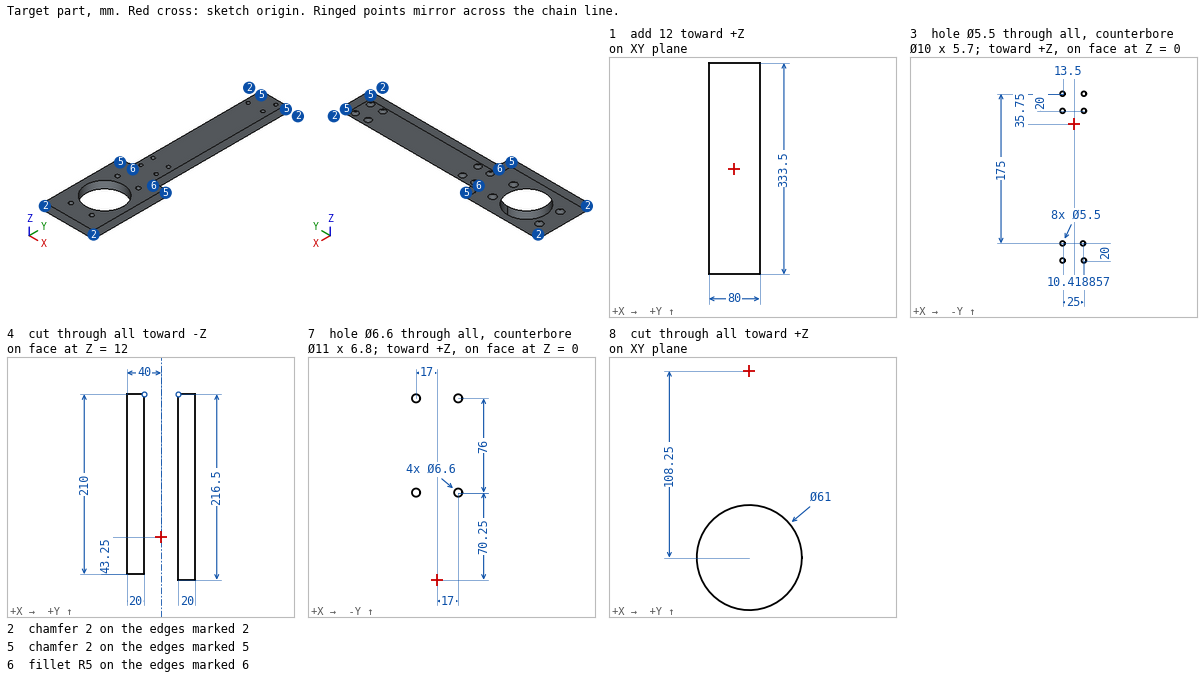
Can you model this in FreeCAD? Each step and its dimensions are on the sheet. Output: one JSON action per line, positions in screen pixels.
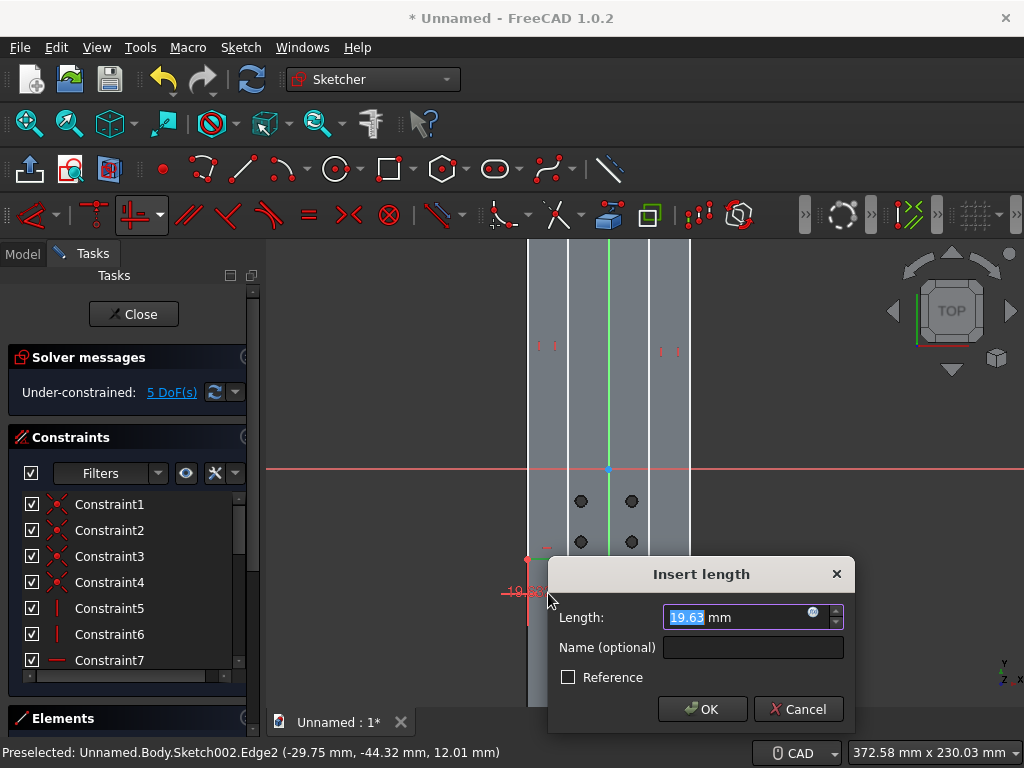
{"action": "type", "text": "20"}
{"action": "key", "text": "Return"}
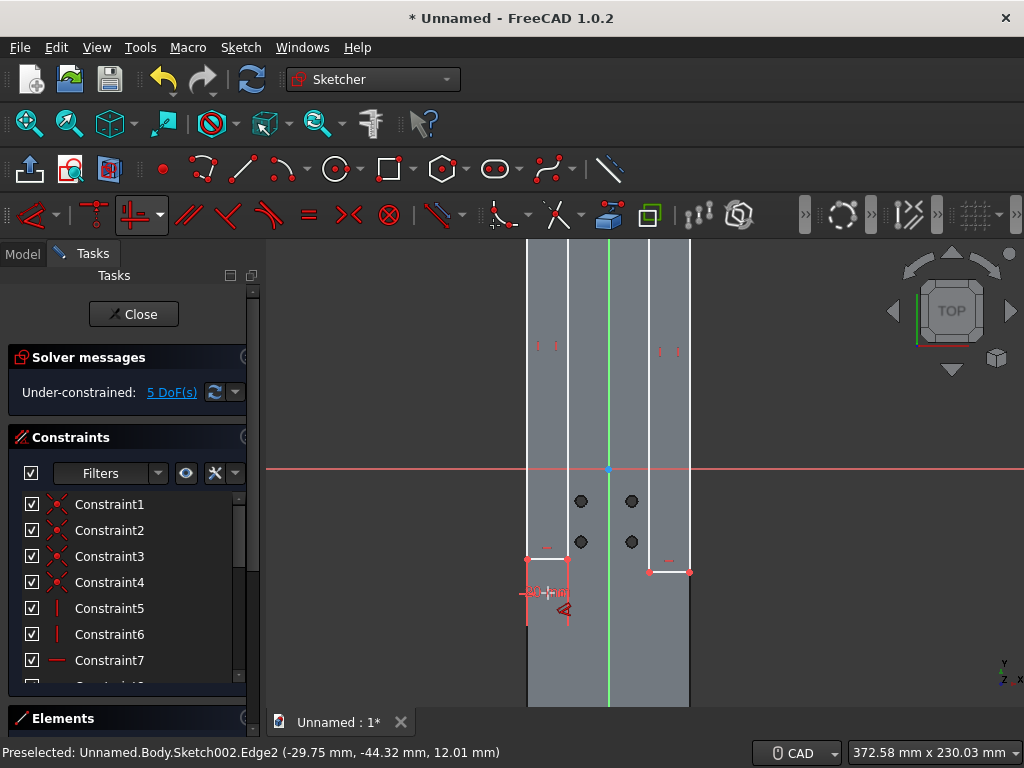
{"action": "left_click", "coordinate": [661, 572]}
{"action": "left_click", "coordinate": [670, 606]}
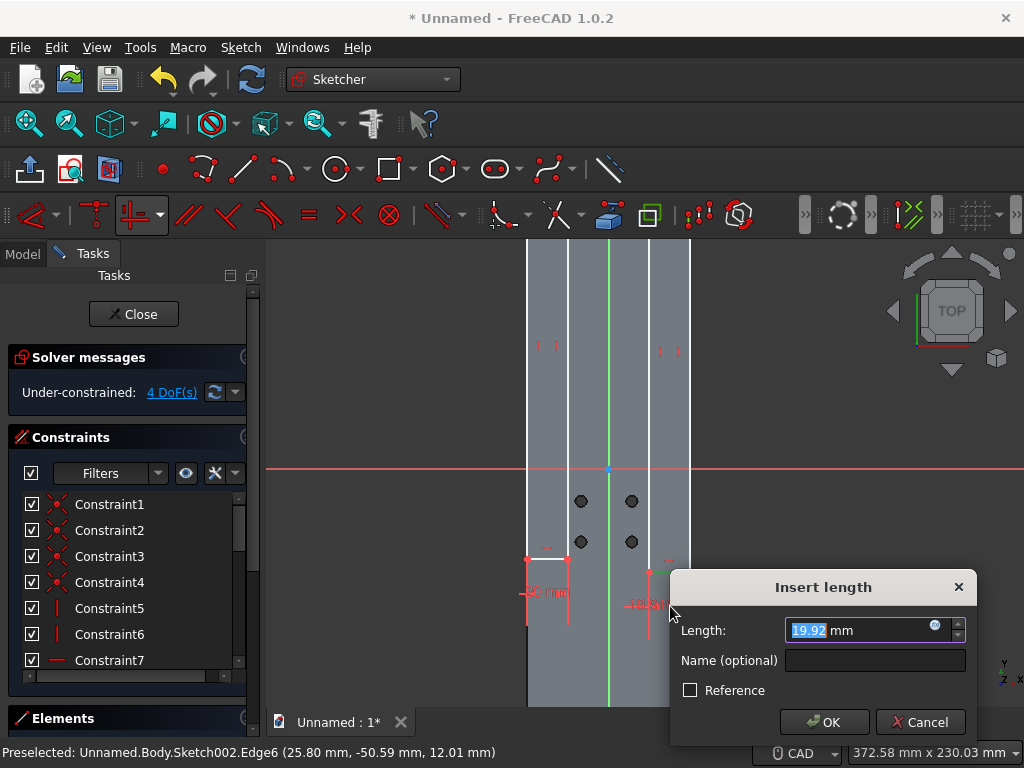
{"action": "type", "text": "20"}
{"action": "key", "text": "Return"}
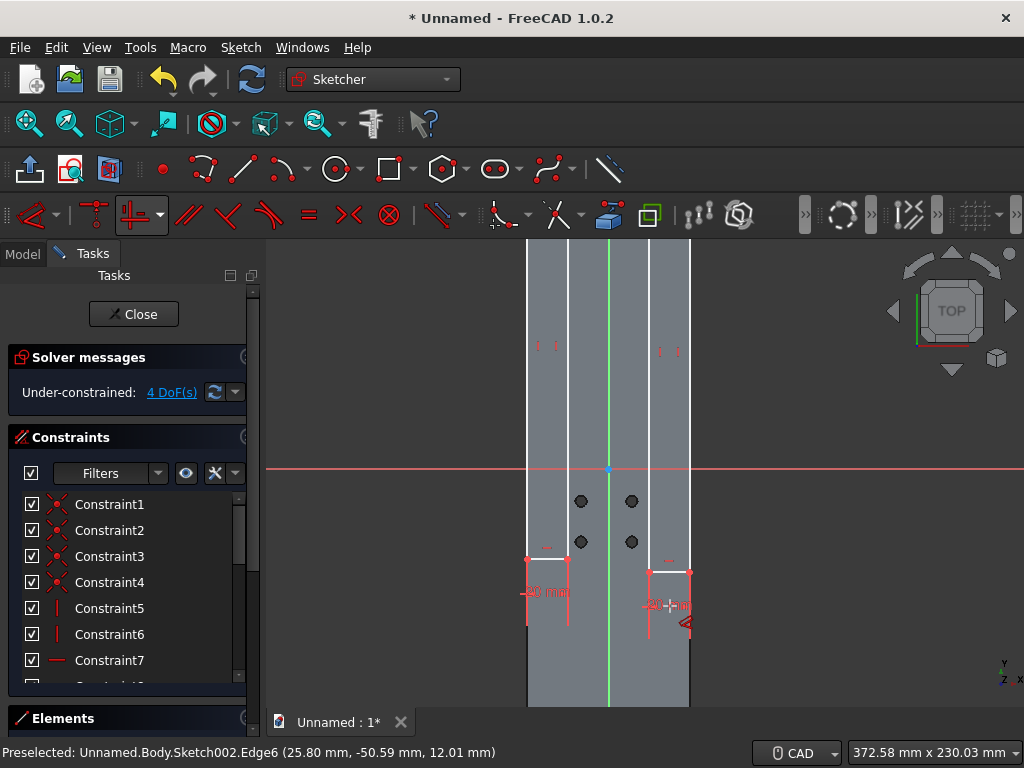
{"action": "left_click", "coordinate": [527, 431]}
{"action": "left_click", "coordinate": [493, 413]}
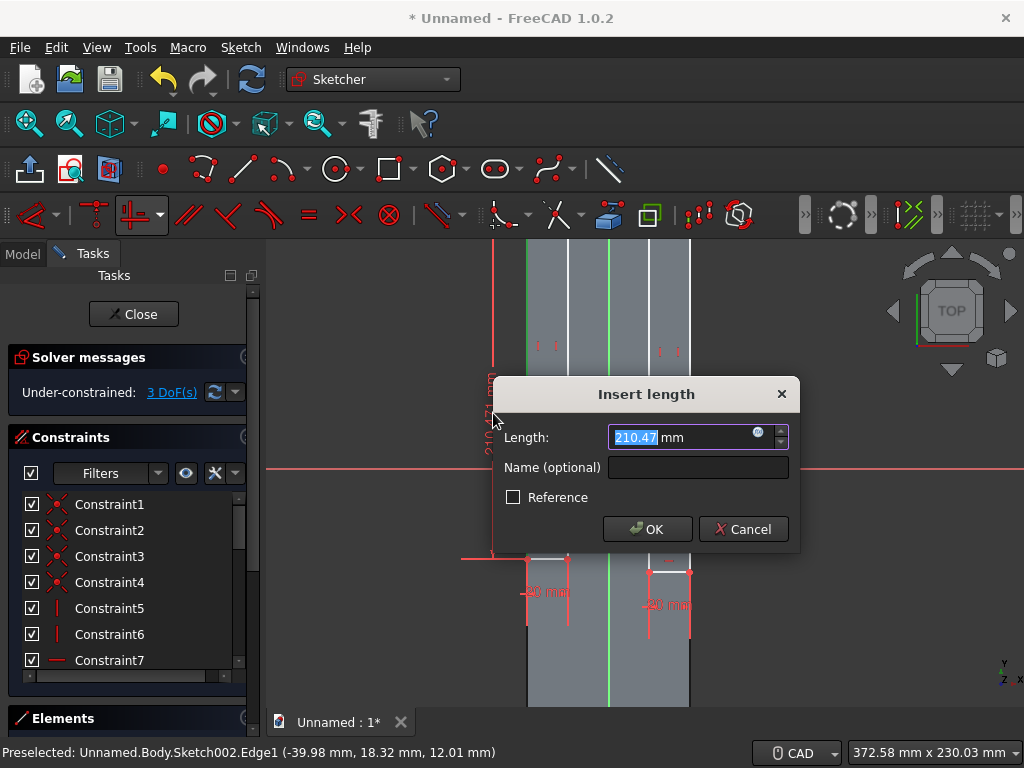
{"action": "type", "text": "210"}
{"action": "key", "text": "Return"}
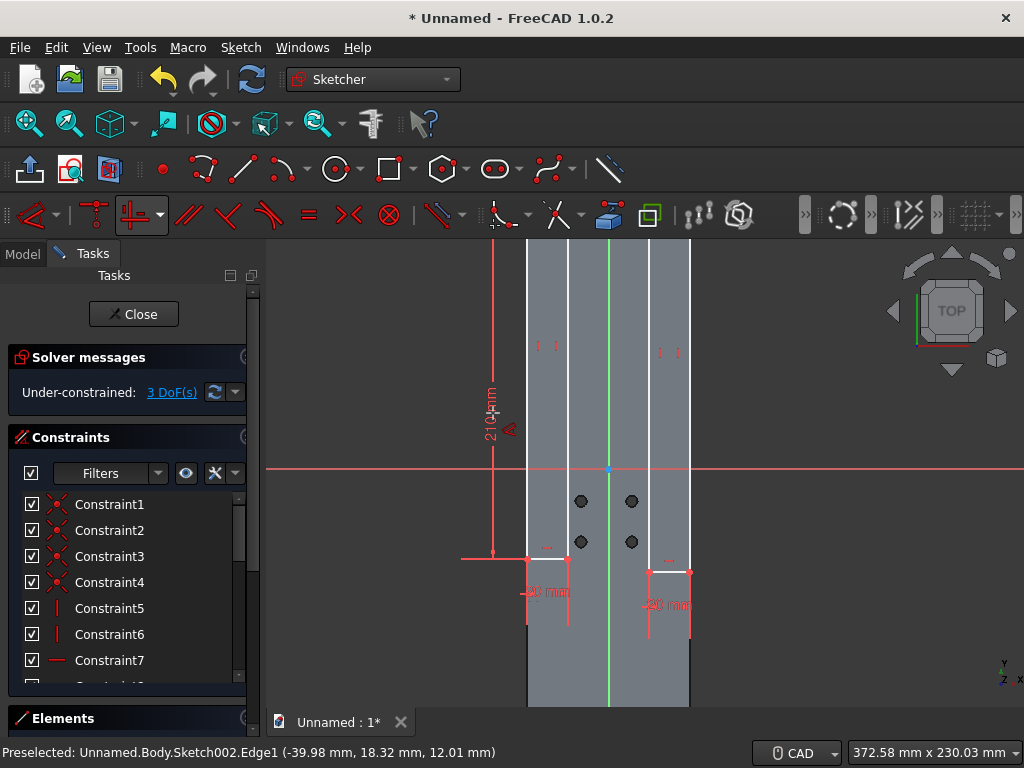
{"action": "scroll", "coordinate": [511, 679], "scroll_direction": "down", "scroll_amount": 2}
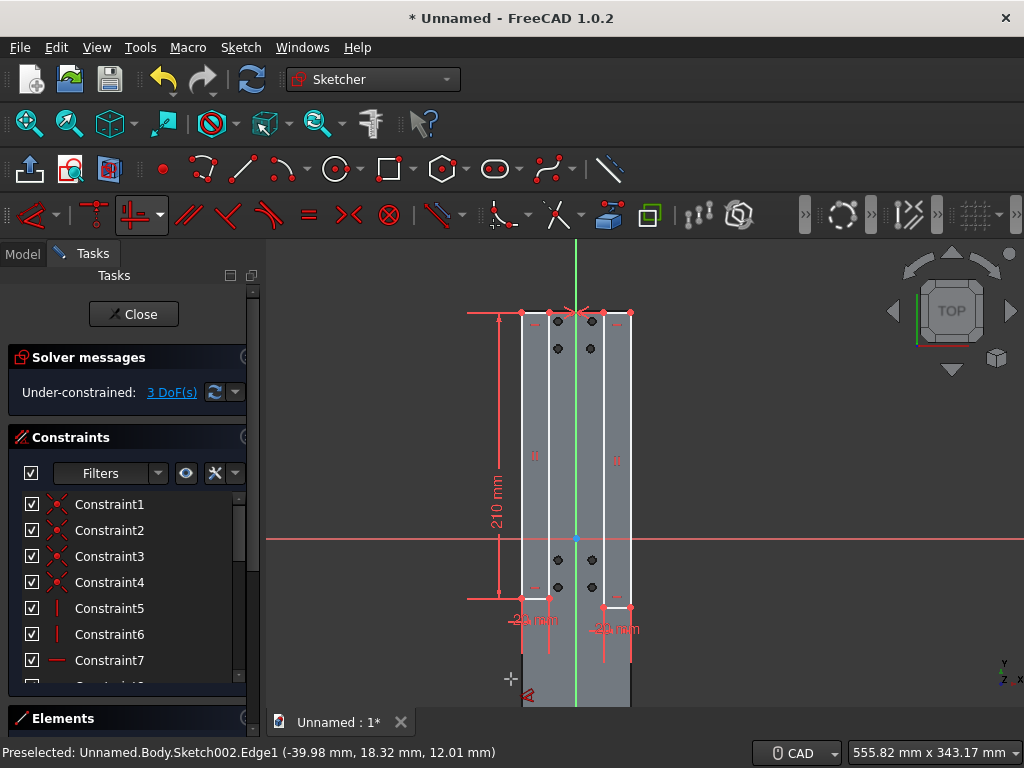
{"action": "left_click", "coordinate": [522, 313]}
{"action": "left_click", "coordinate": [549, 279]}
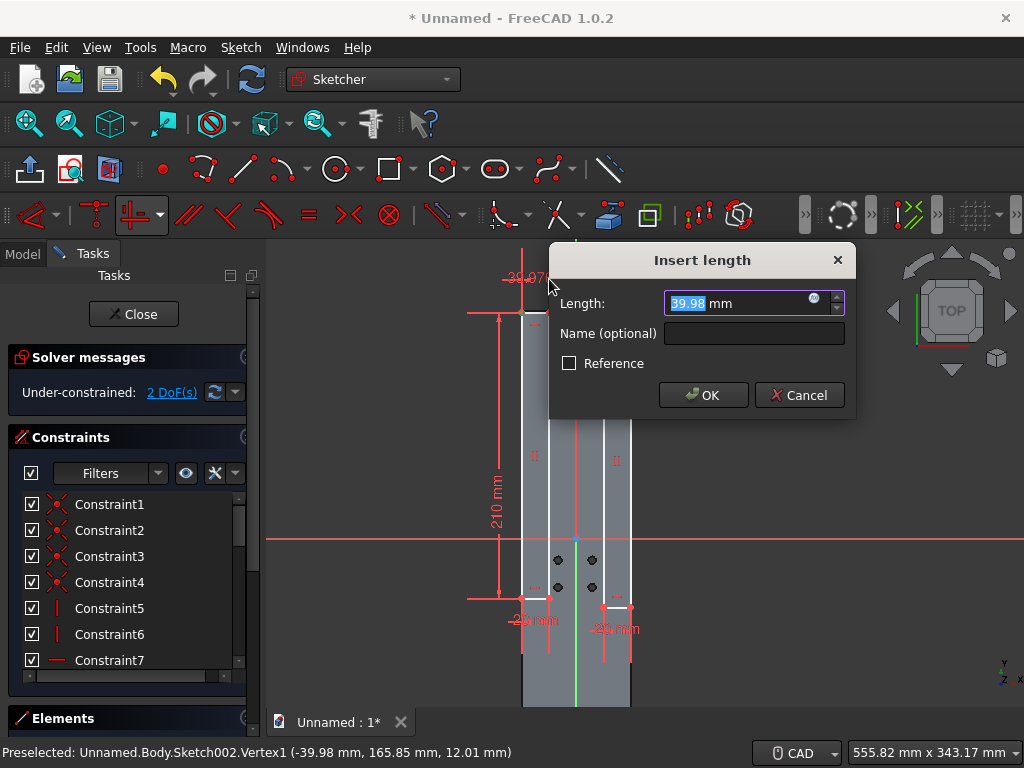
{"action": "type", "text": "40"}
{"action": "key", "text": "Return"}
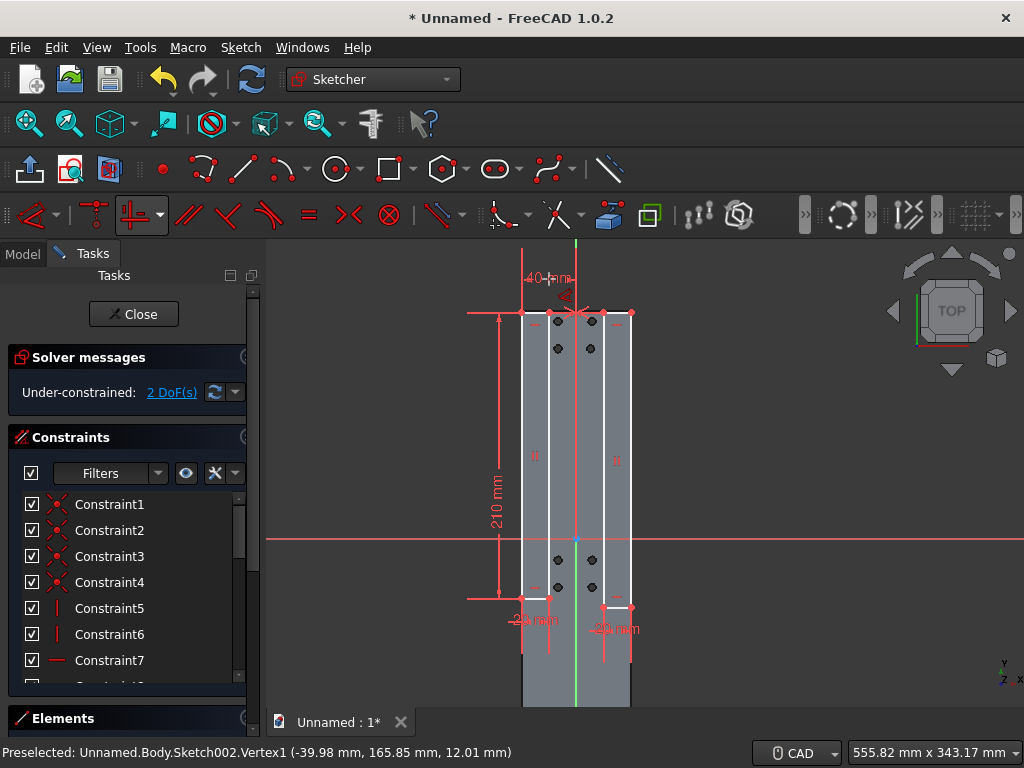
{"action": "left_click", "coordinate": [604, 401]}
{"action": "left_click", "coordinate": [662, 460]}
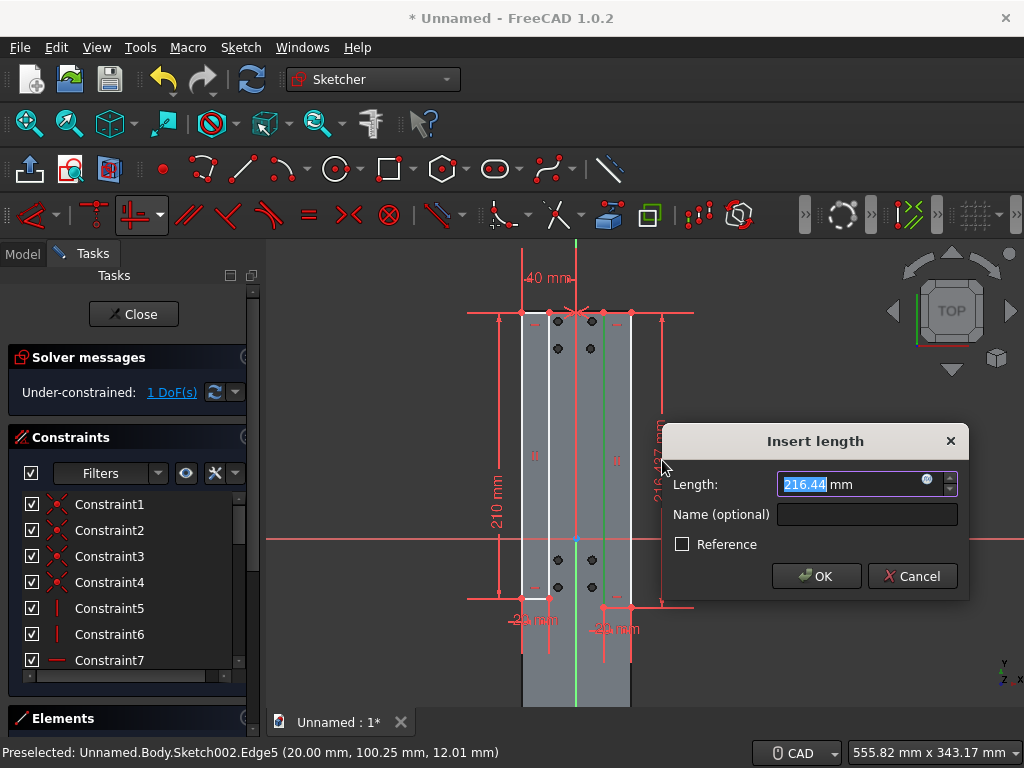
{"action": "type", "text": "216.5"}
{"action": "key", "text": "Return"}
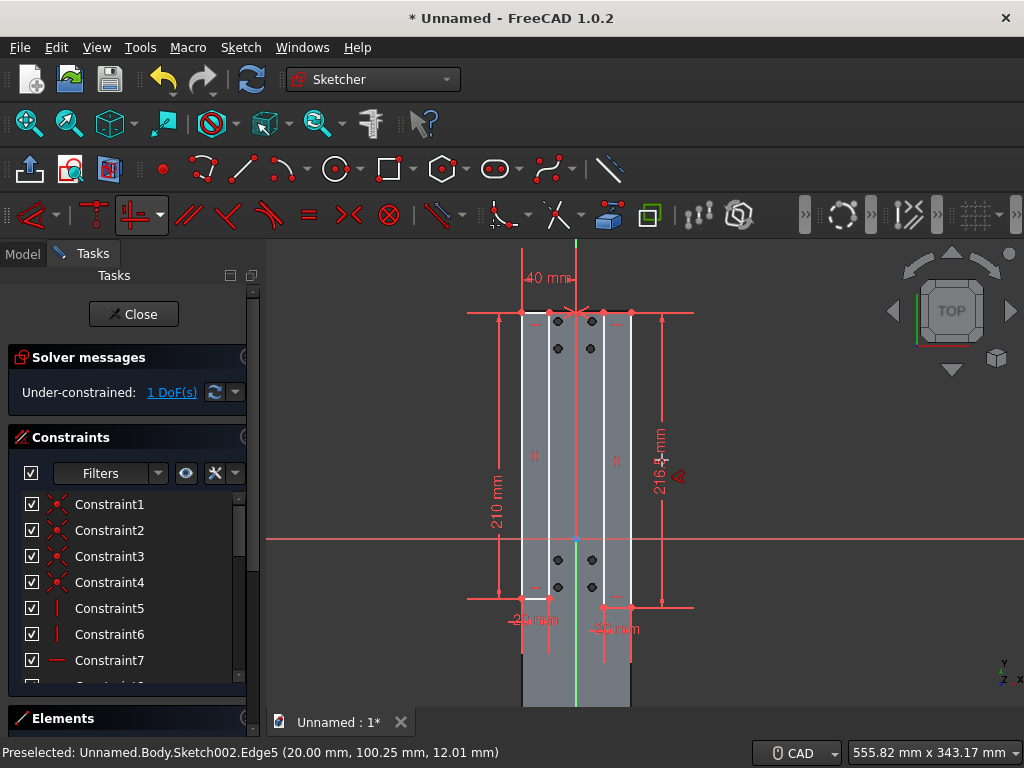
{"action": "left_click", "coordinate": [522, 599]}
{"action": "left_click", "coordinate": [488, 569]}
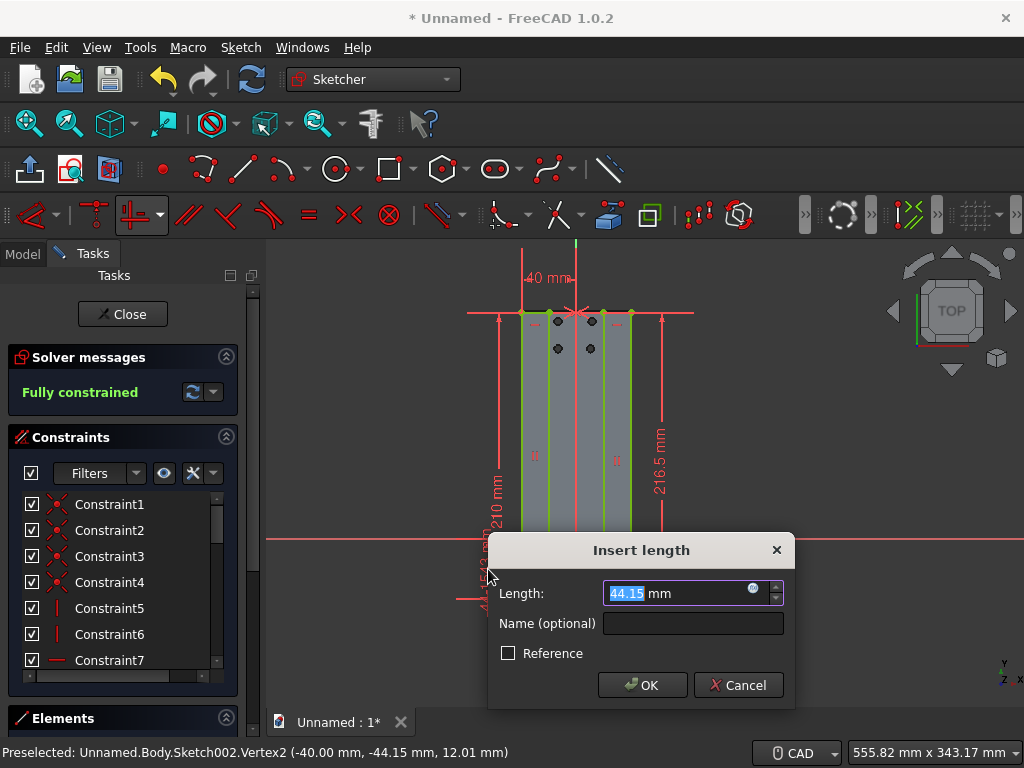
{"action": "type", "text": "43.25"}
{"action": "key", "text": "Return"}
{"action": "key", "text": "Escape"}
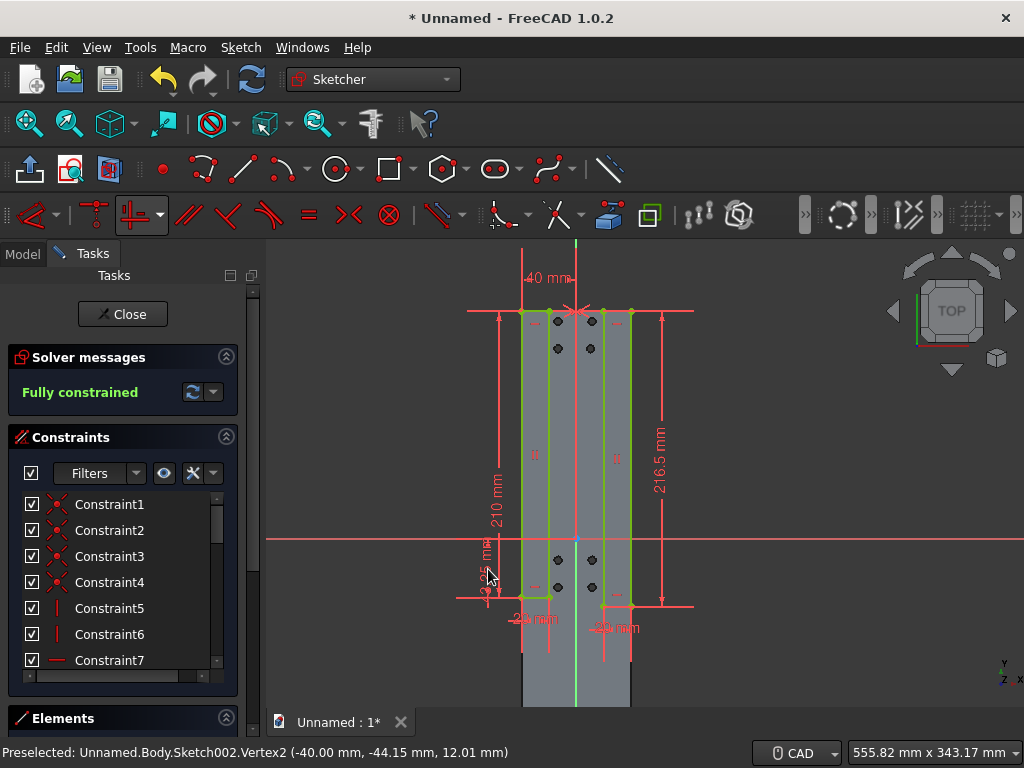
{"action": "left_click", "coordinate": [123, 314]}